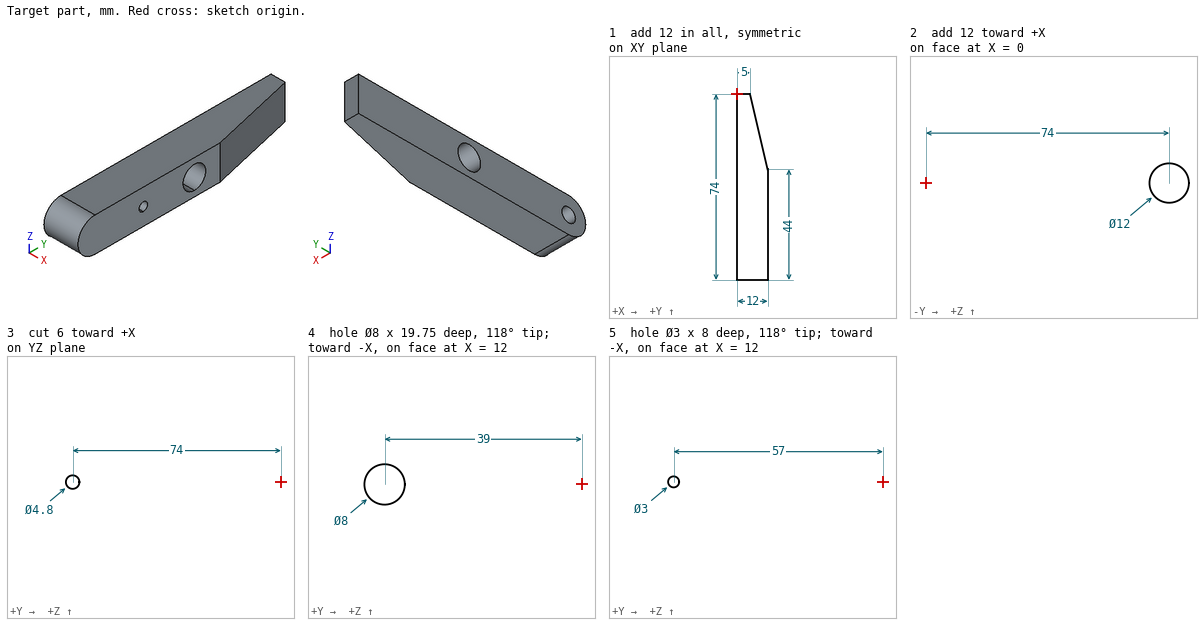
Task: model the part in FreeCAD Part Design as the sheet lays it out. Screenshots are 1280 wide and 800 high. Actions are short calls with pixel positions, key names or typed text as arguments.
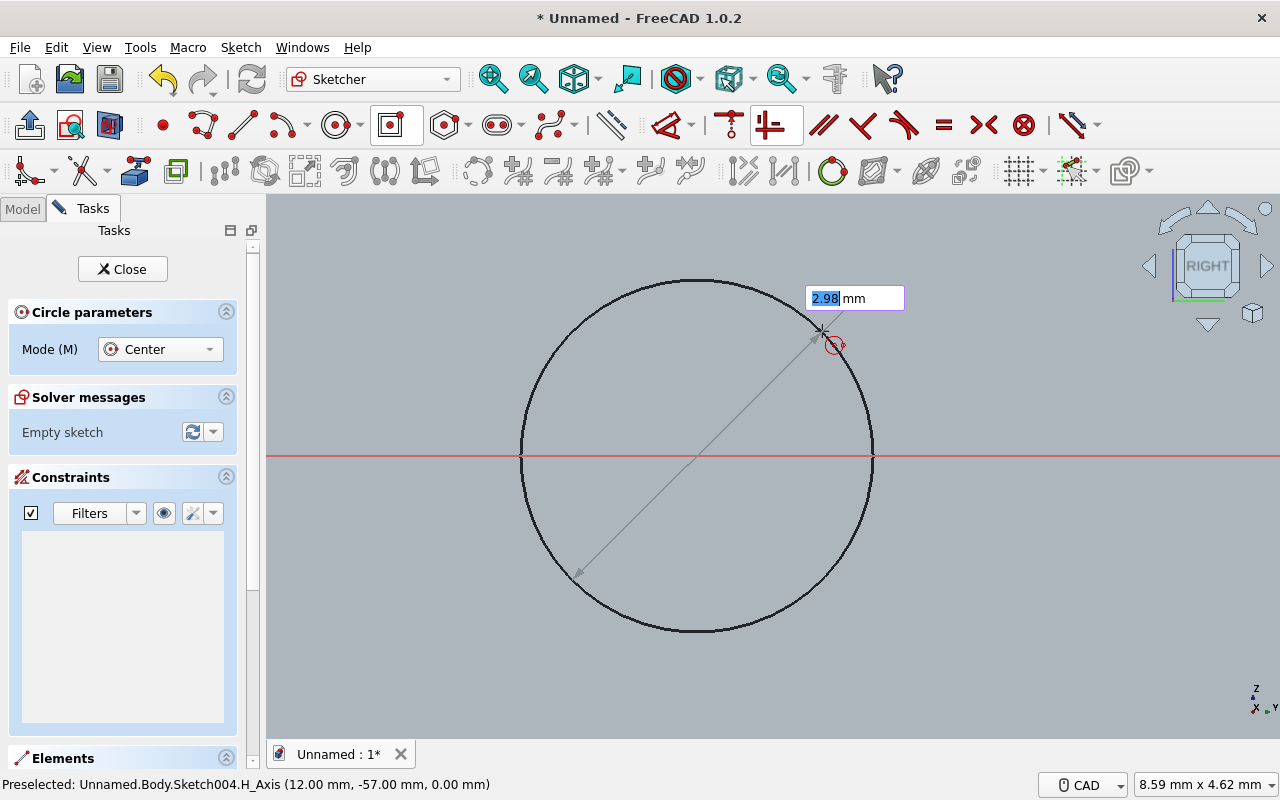
text(3)
key(Return)
key(Escape)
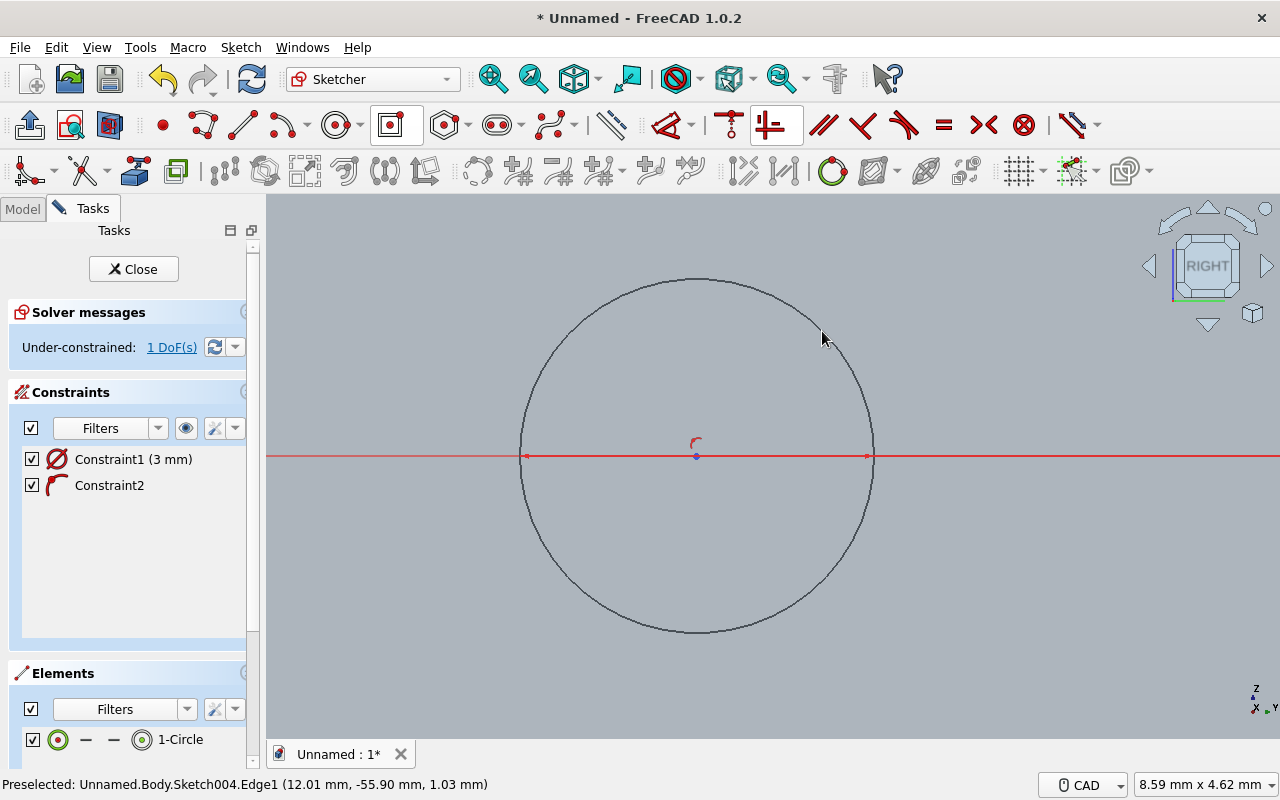
key(d)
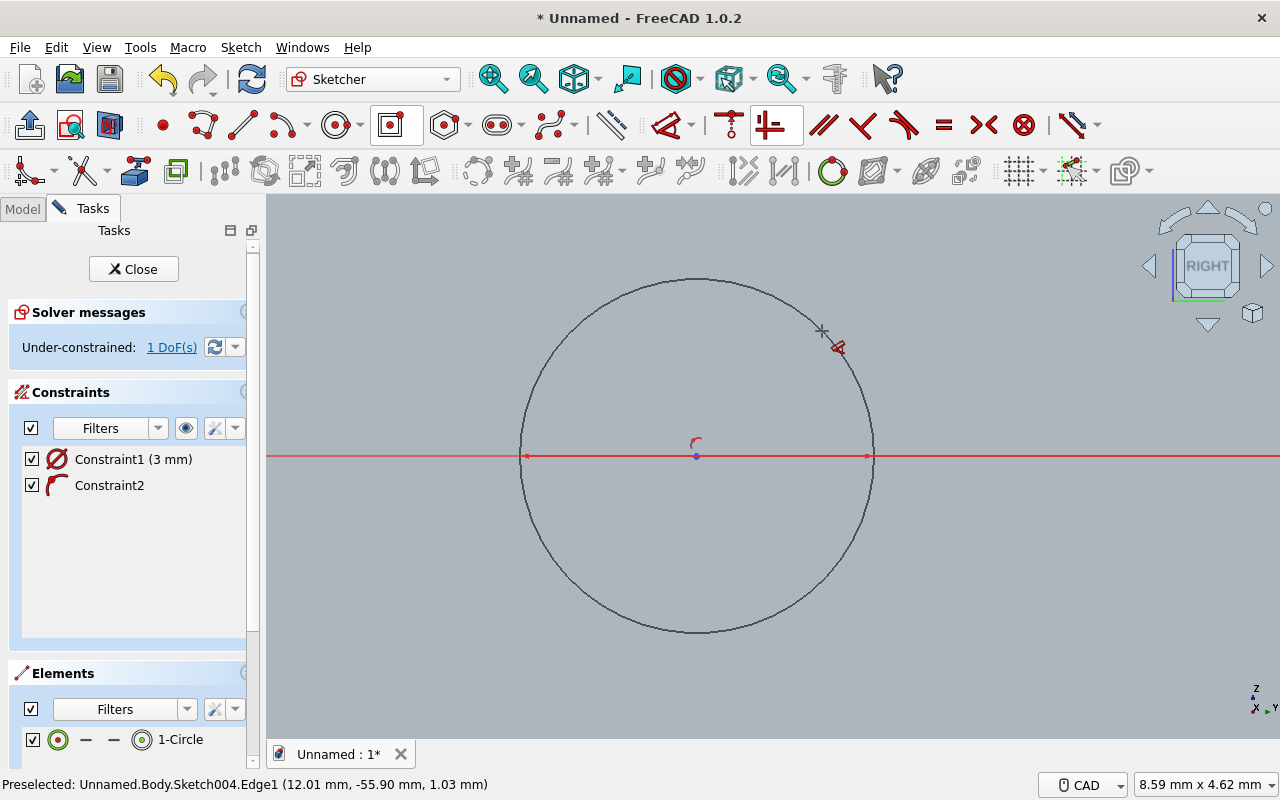
click(697, 456)
click(906, 490)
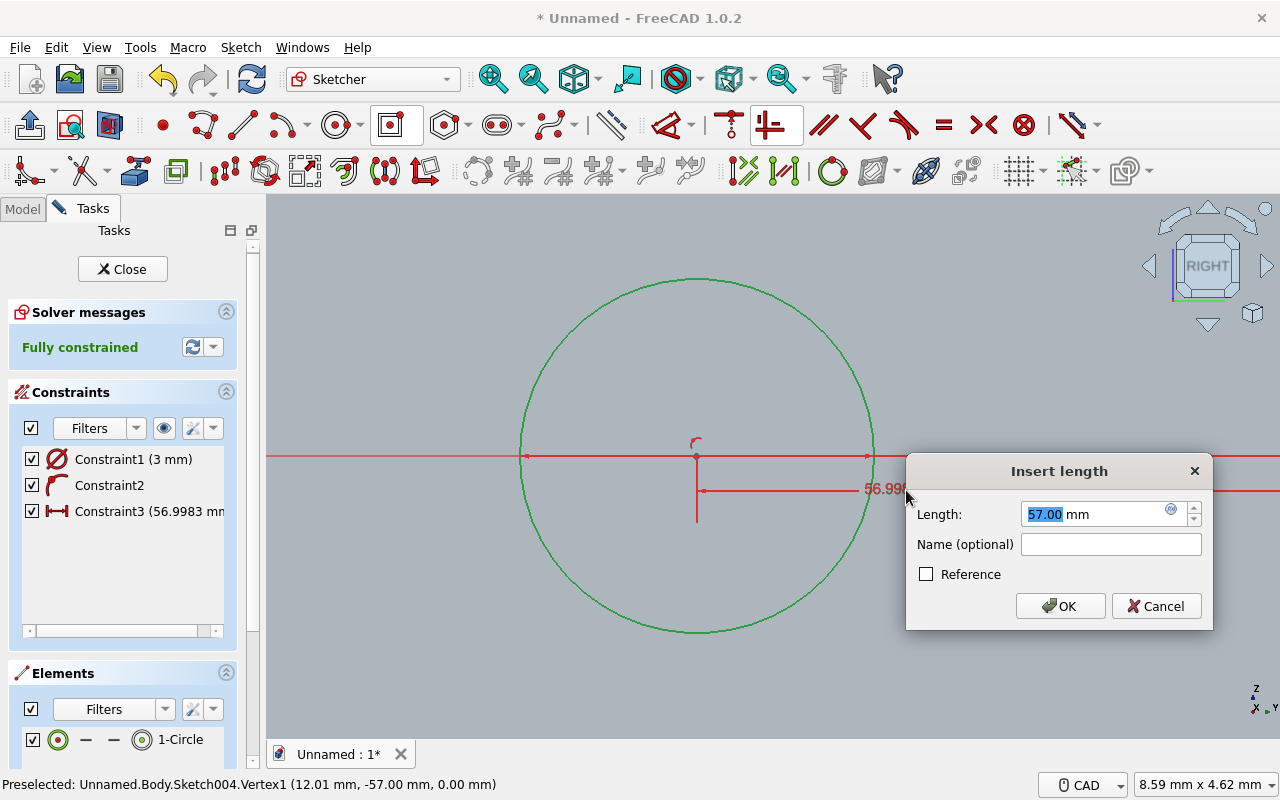
text(57)
key(Return)
key(Escape)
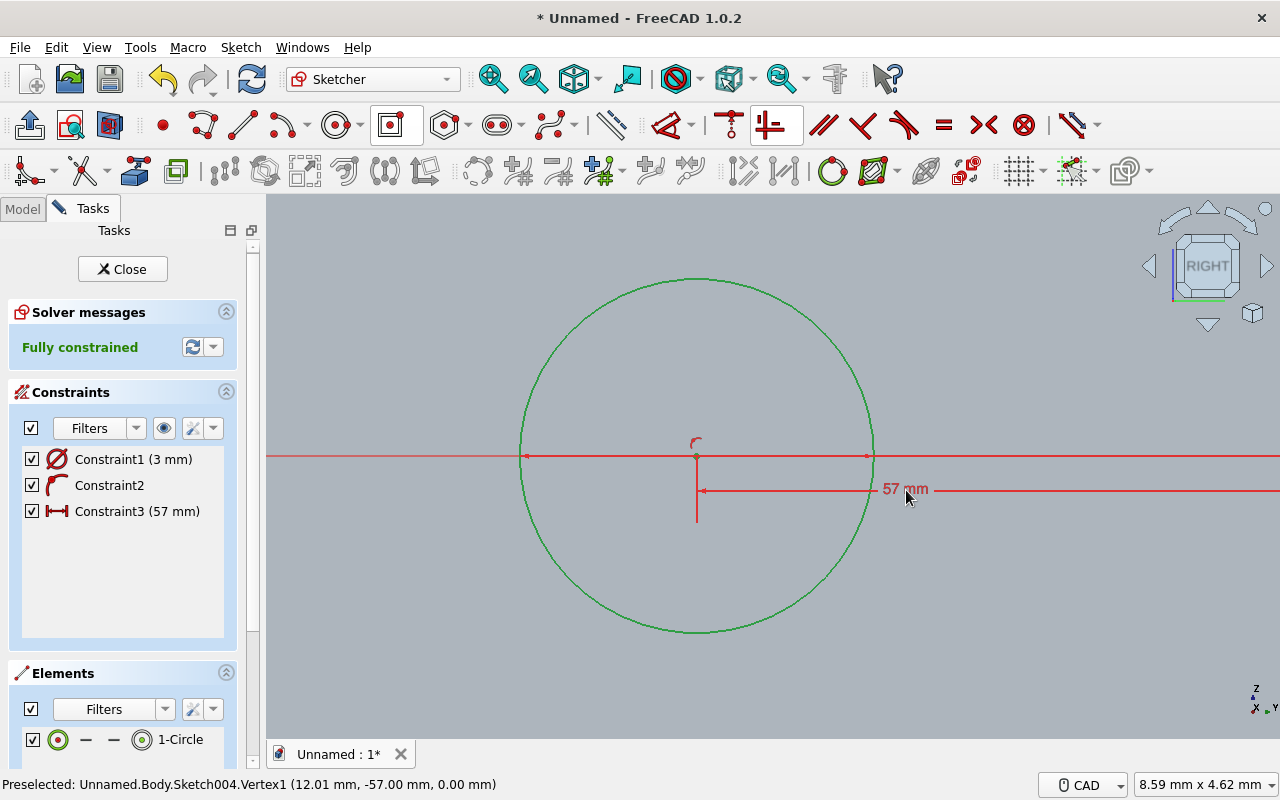
click(123, 269)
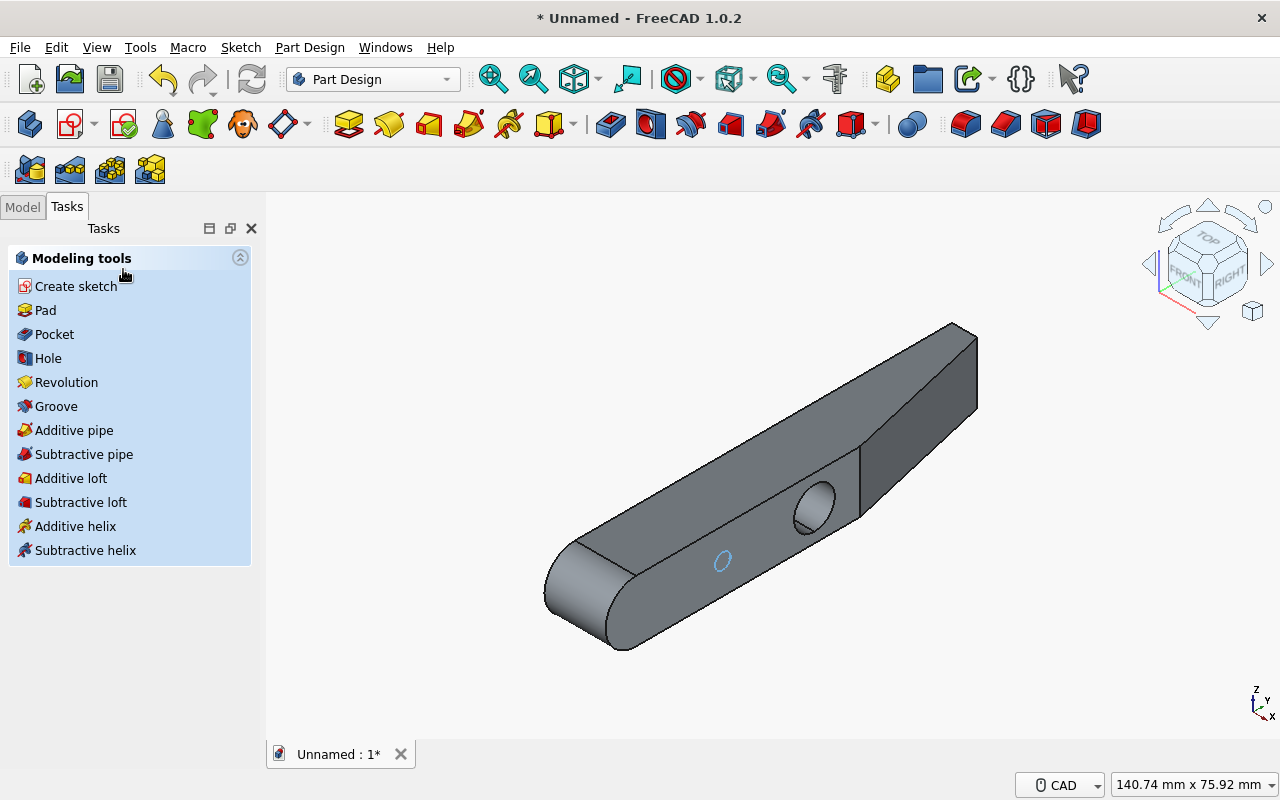
click(652, 124)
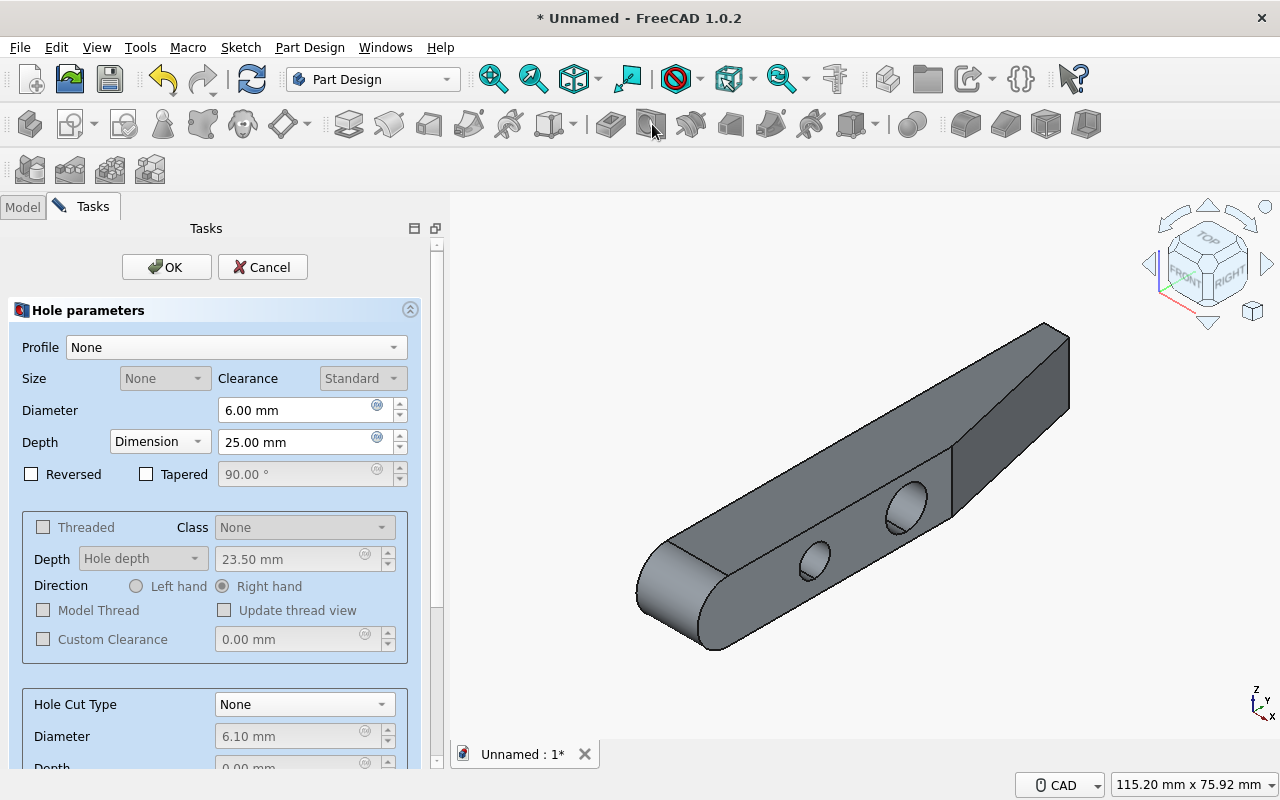
triple_click(305, 410)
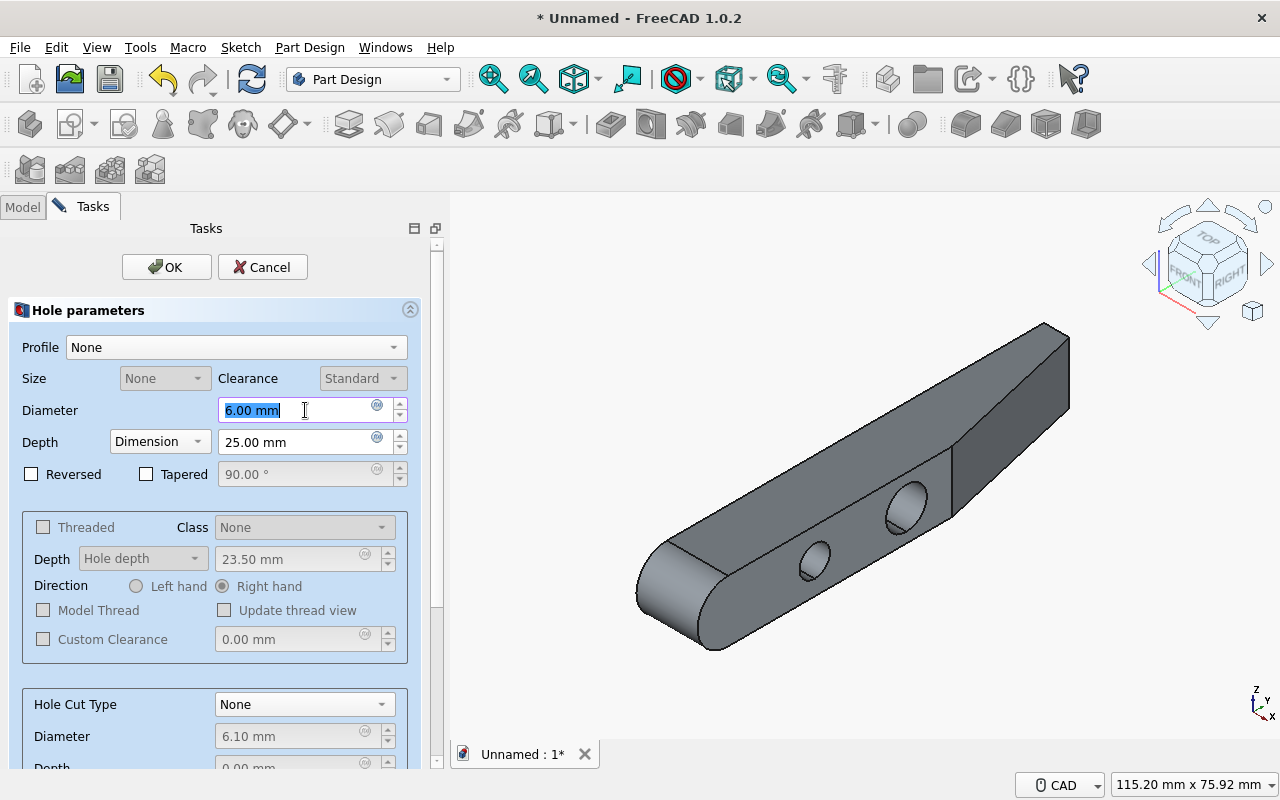
text(3)
key(Tab)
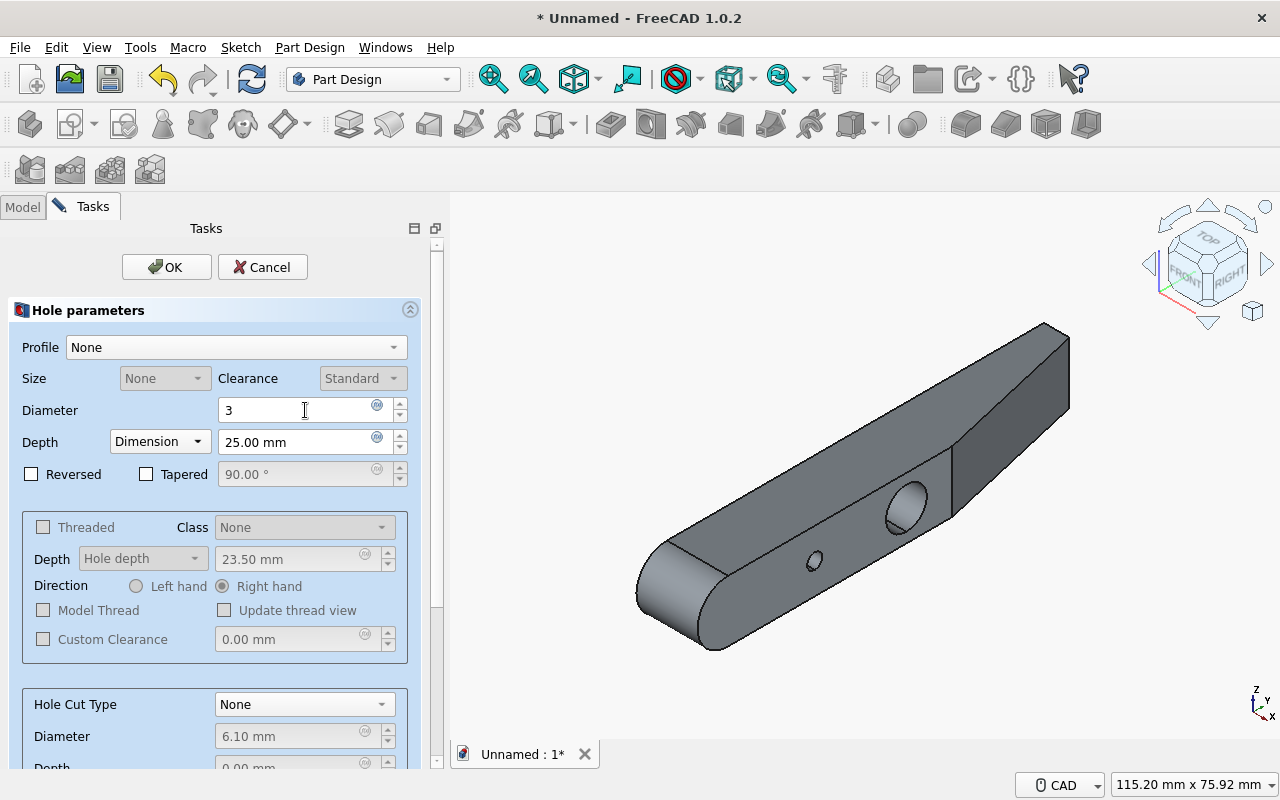
triple_click(305, 442)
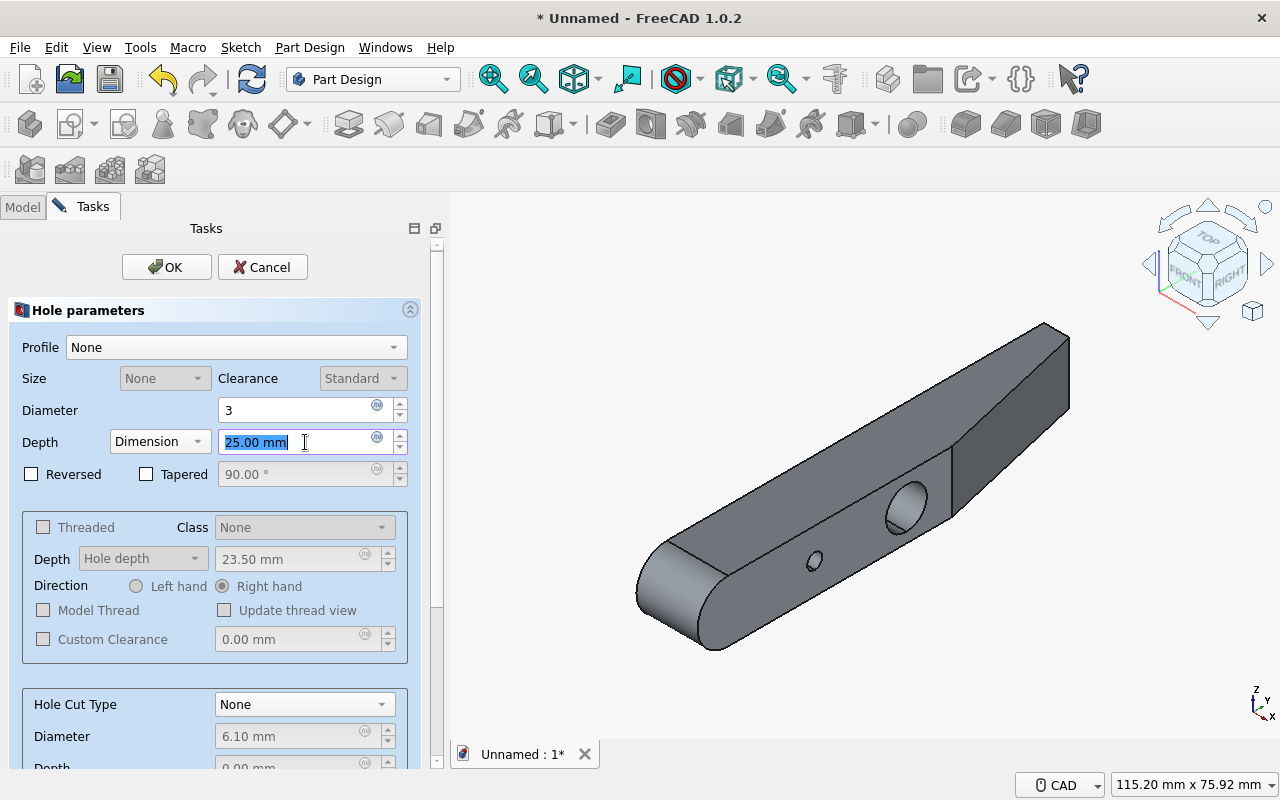
text(8)
key(Tab)